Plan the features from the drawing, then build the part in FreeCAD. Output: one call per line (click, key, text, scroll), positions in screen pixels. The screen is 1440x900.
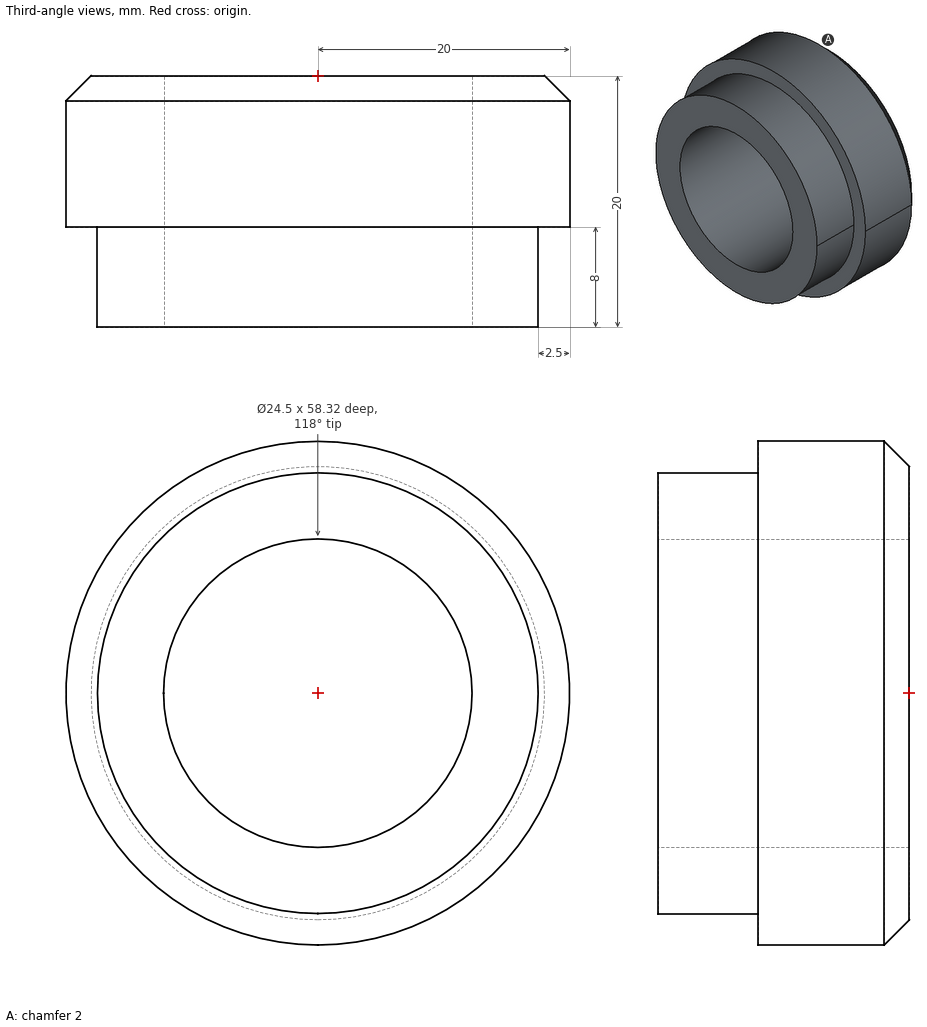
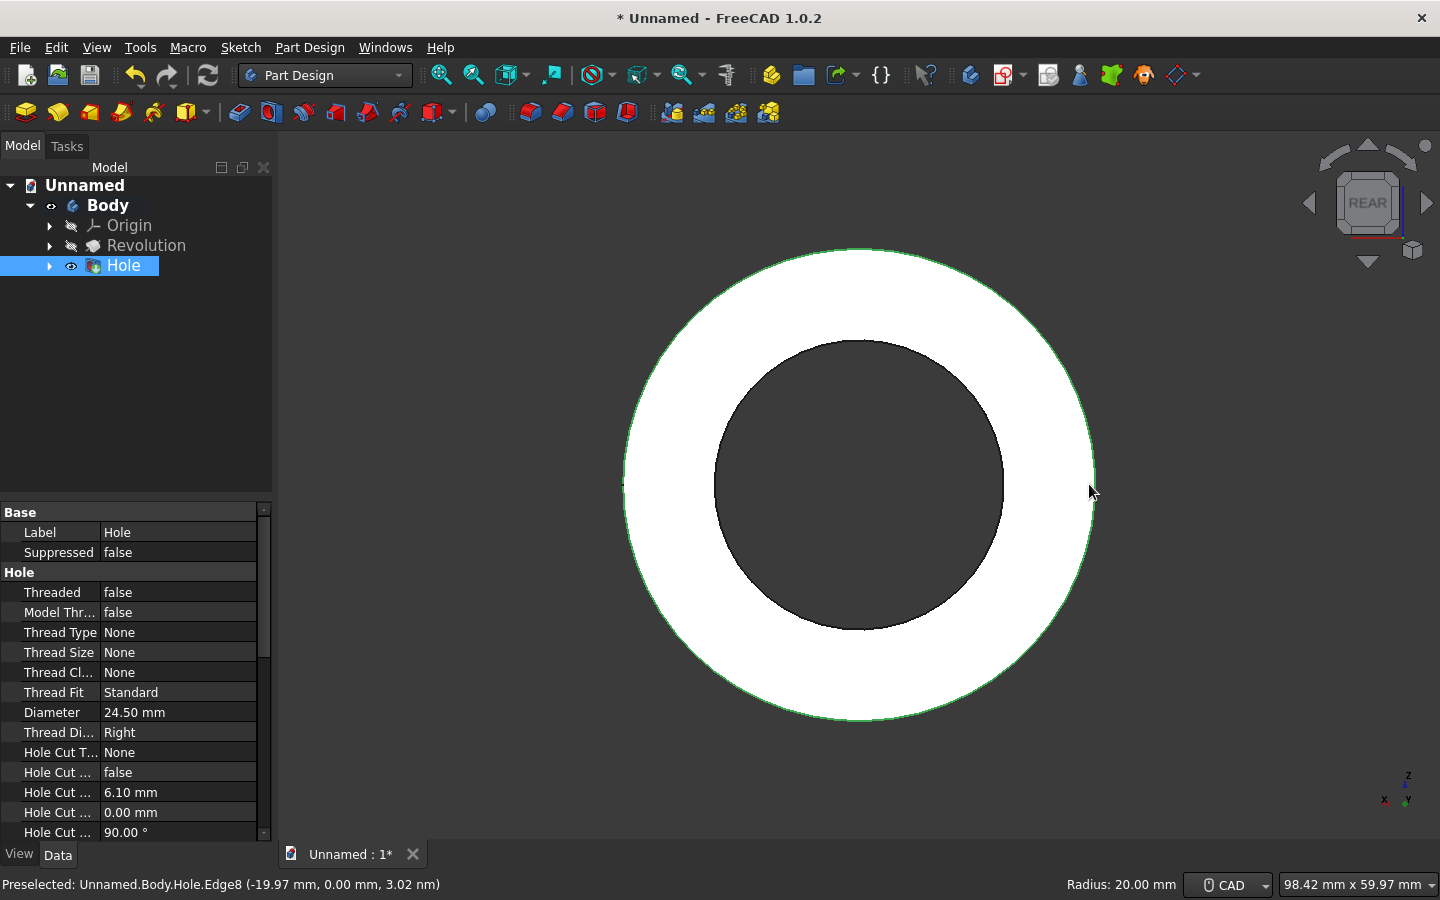
click(564, 112)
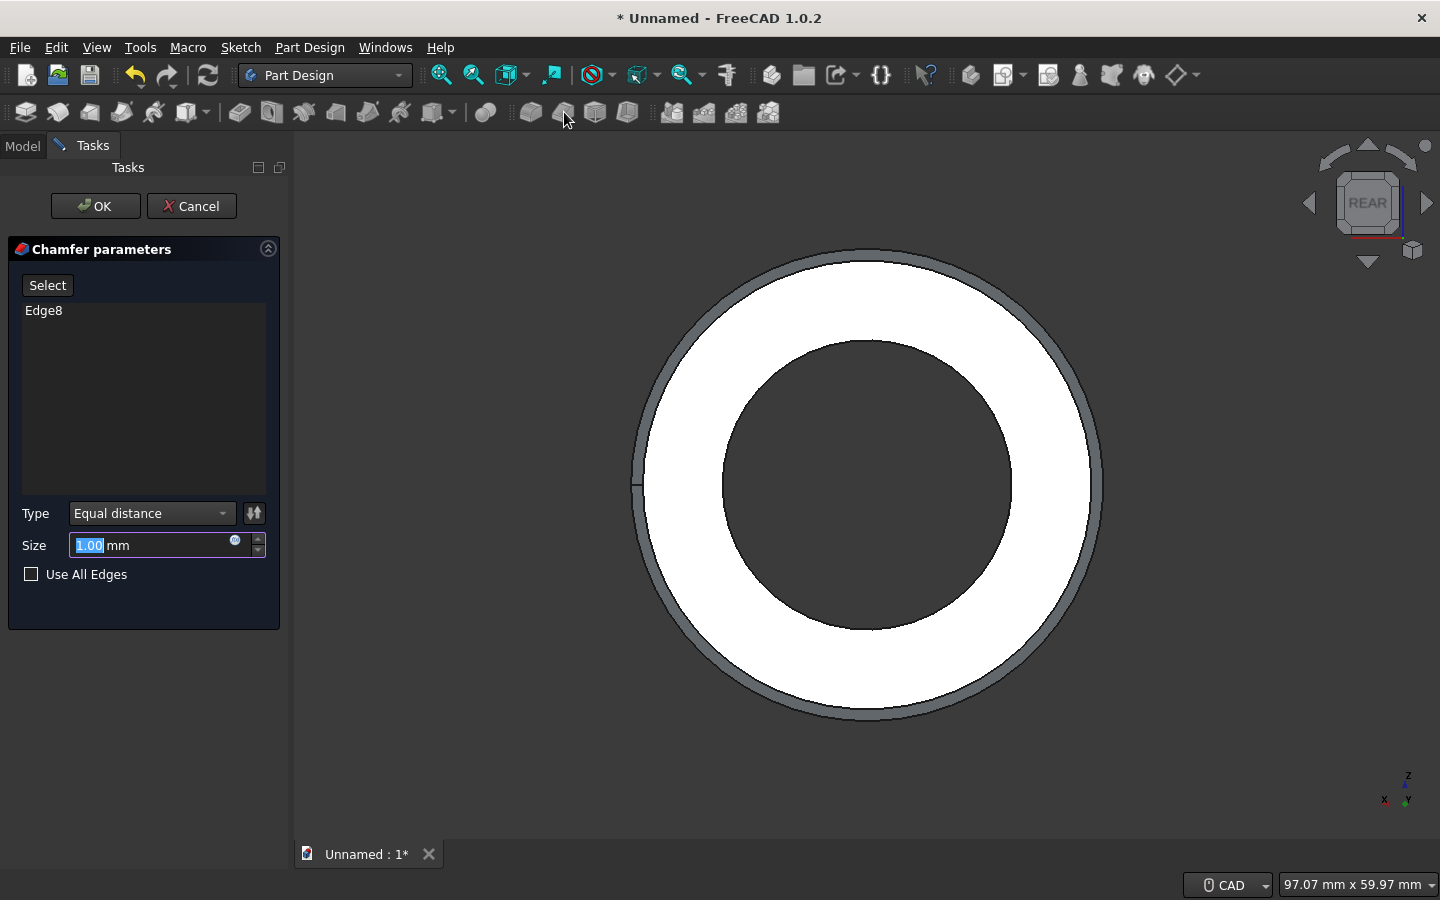
text(2)
key(Tab)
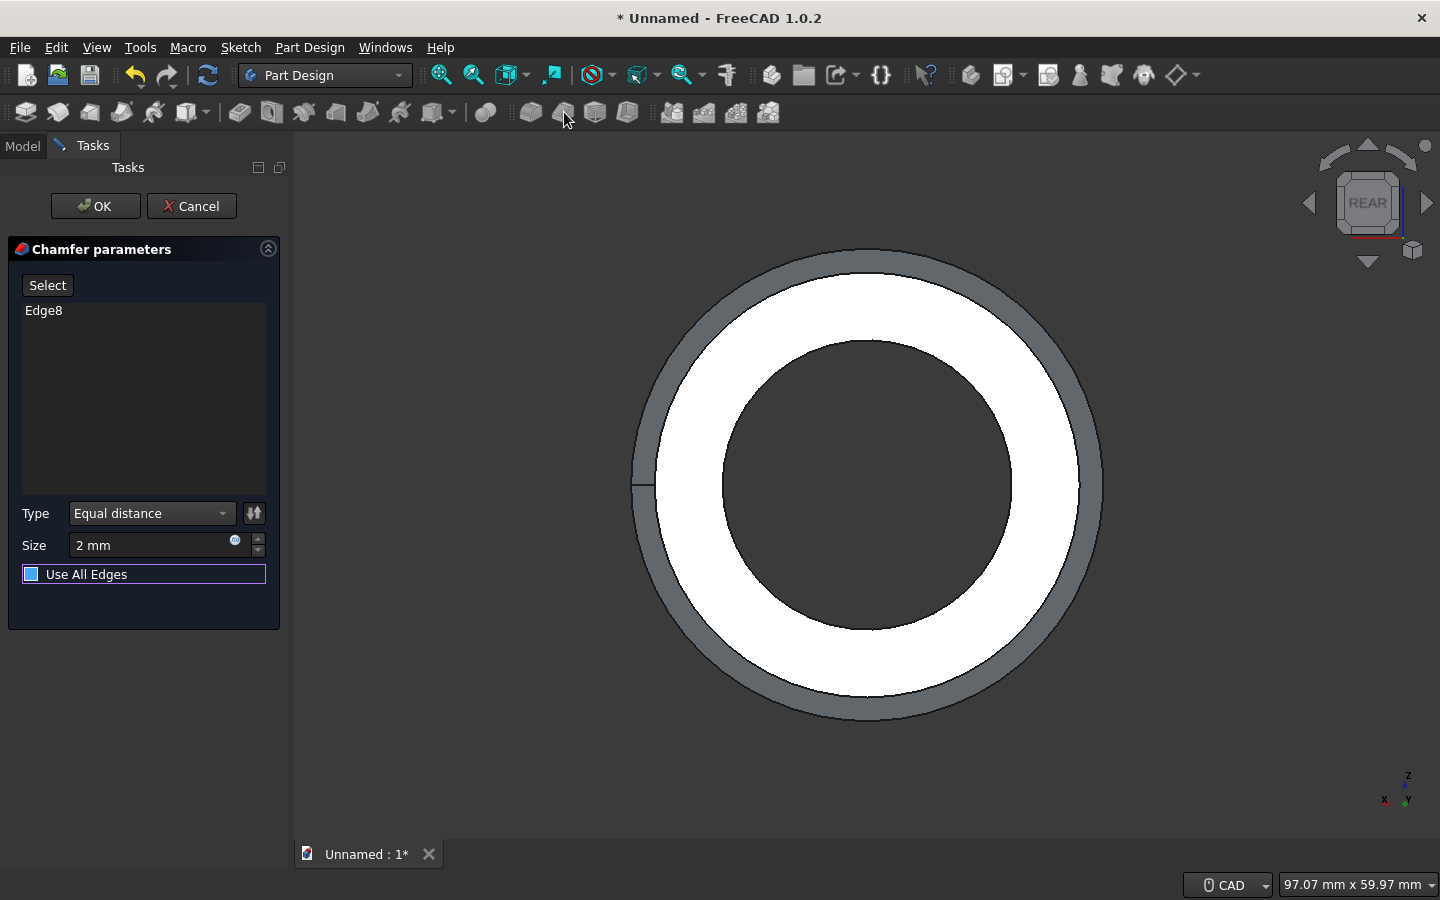
click(96, 206)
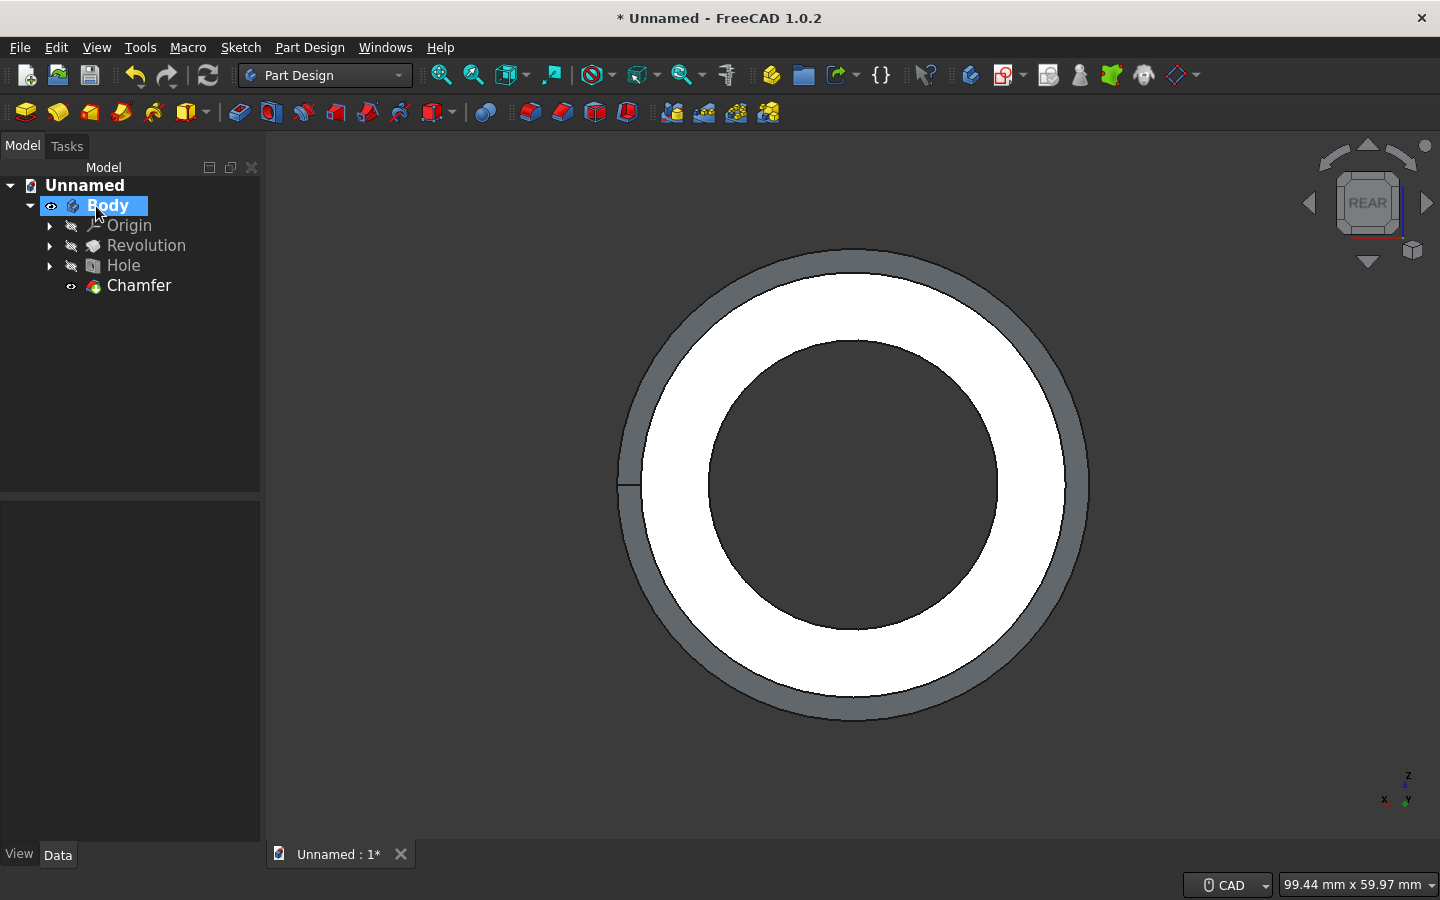
key(0)